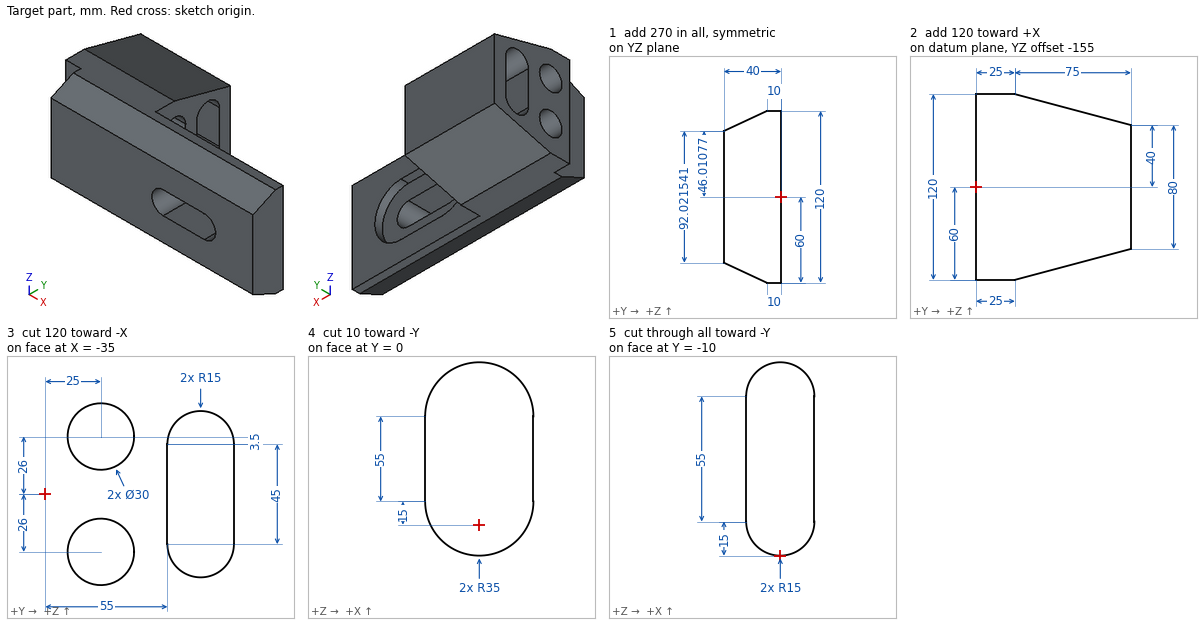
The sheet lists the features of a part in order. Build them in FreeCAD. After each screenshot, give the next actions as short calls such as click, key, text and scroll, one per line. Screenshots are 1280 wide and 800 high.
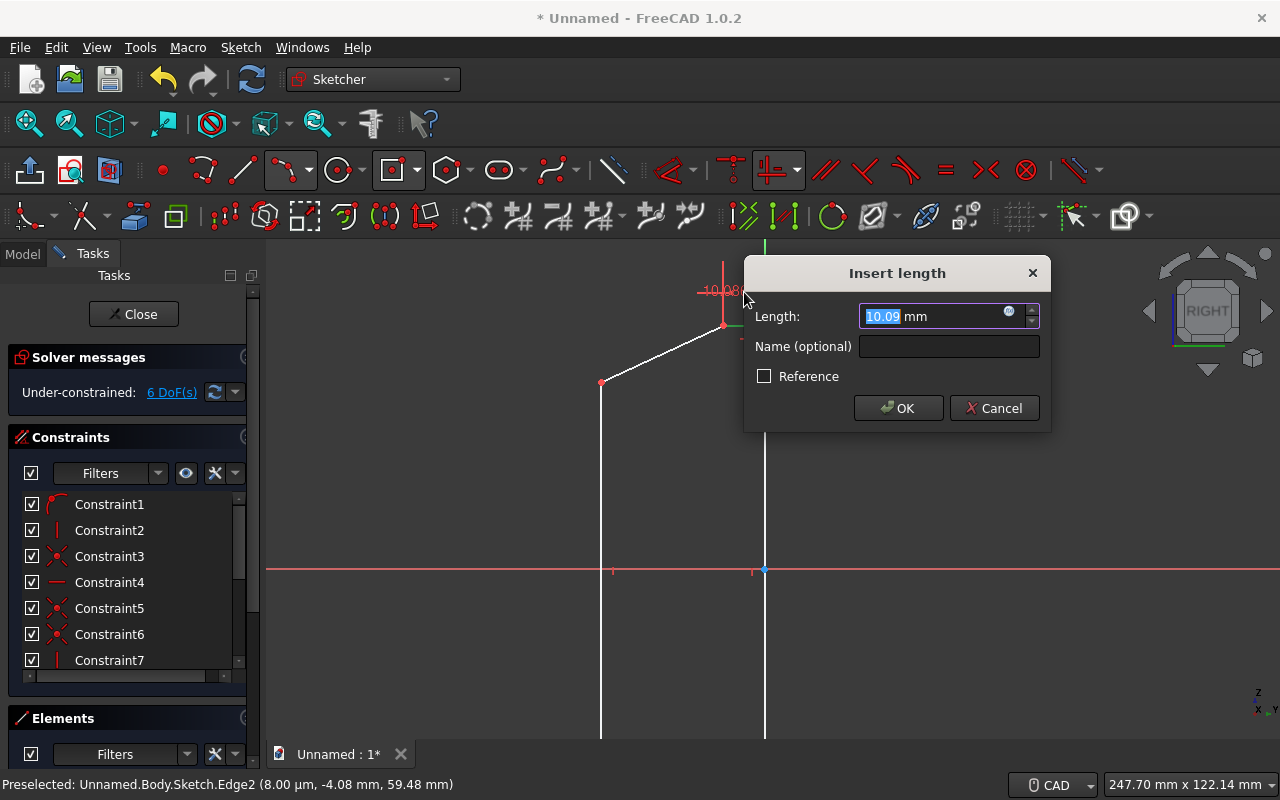
text(10)
key(Return)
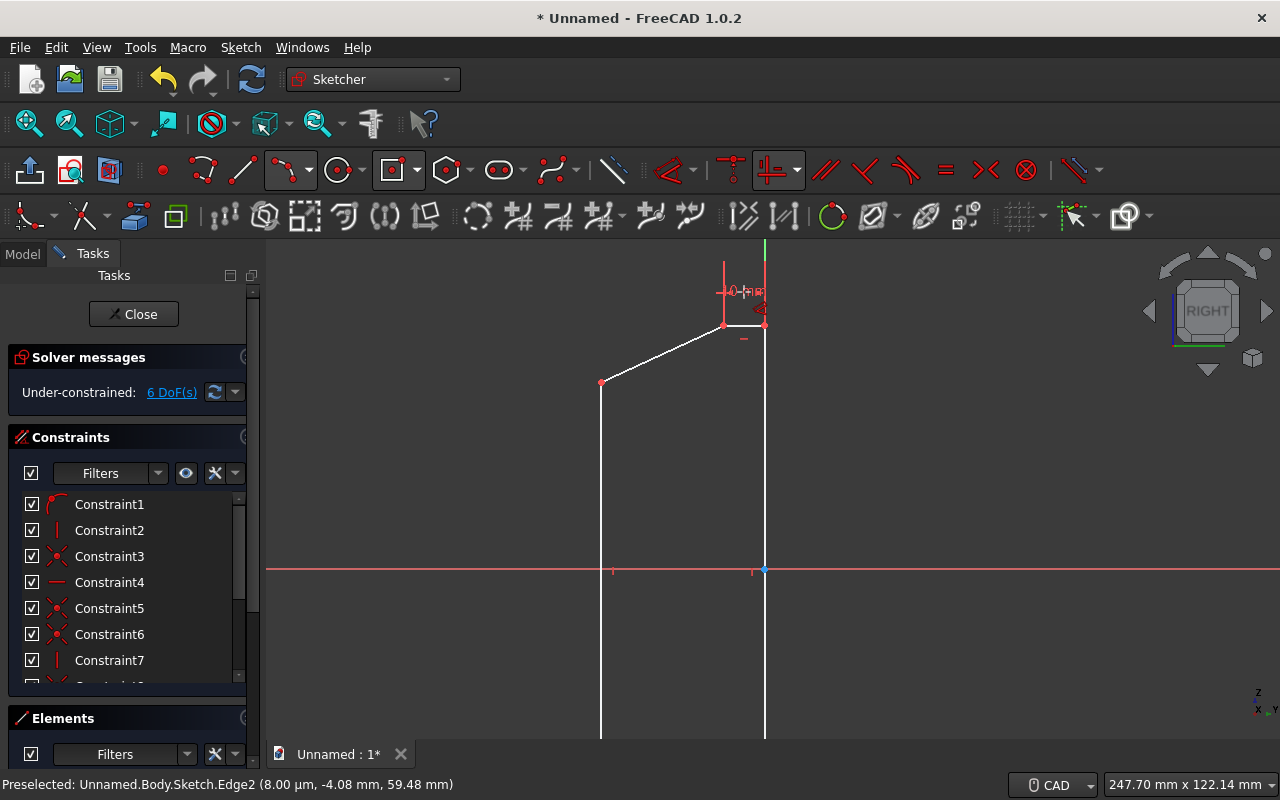
scroll(749, 325, down, 2)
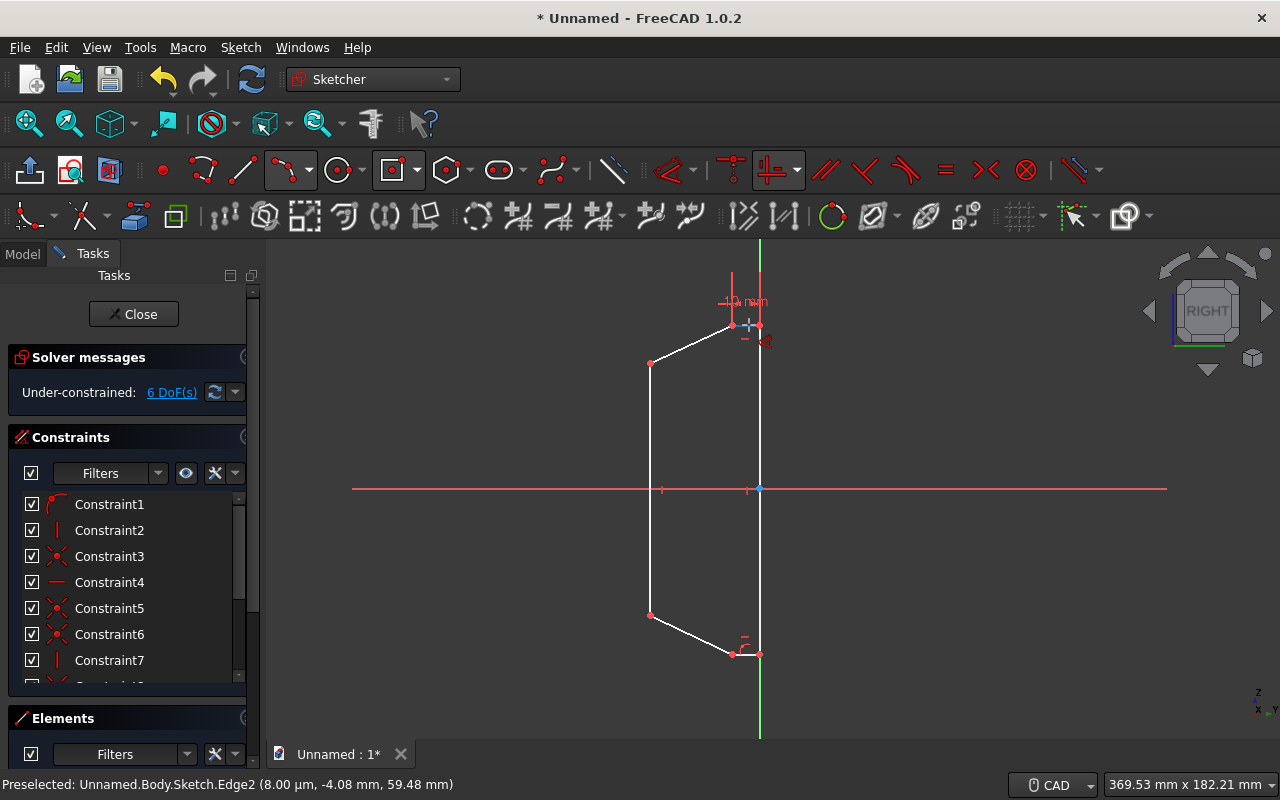
scroll(740, 655, up, 3)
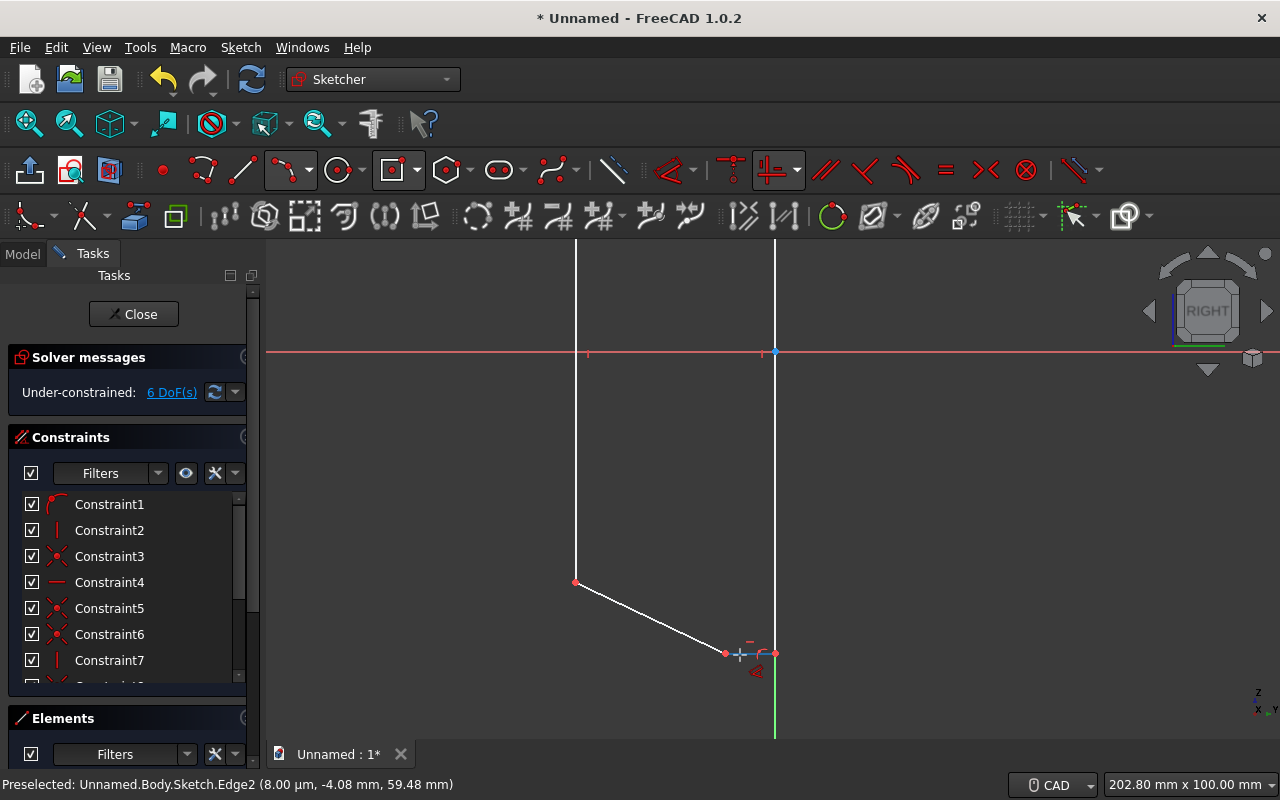
click(740, 654)
click(750, 688)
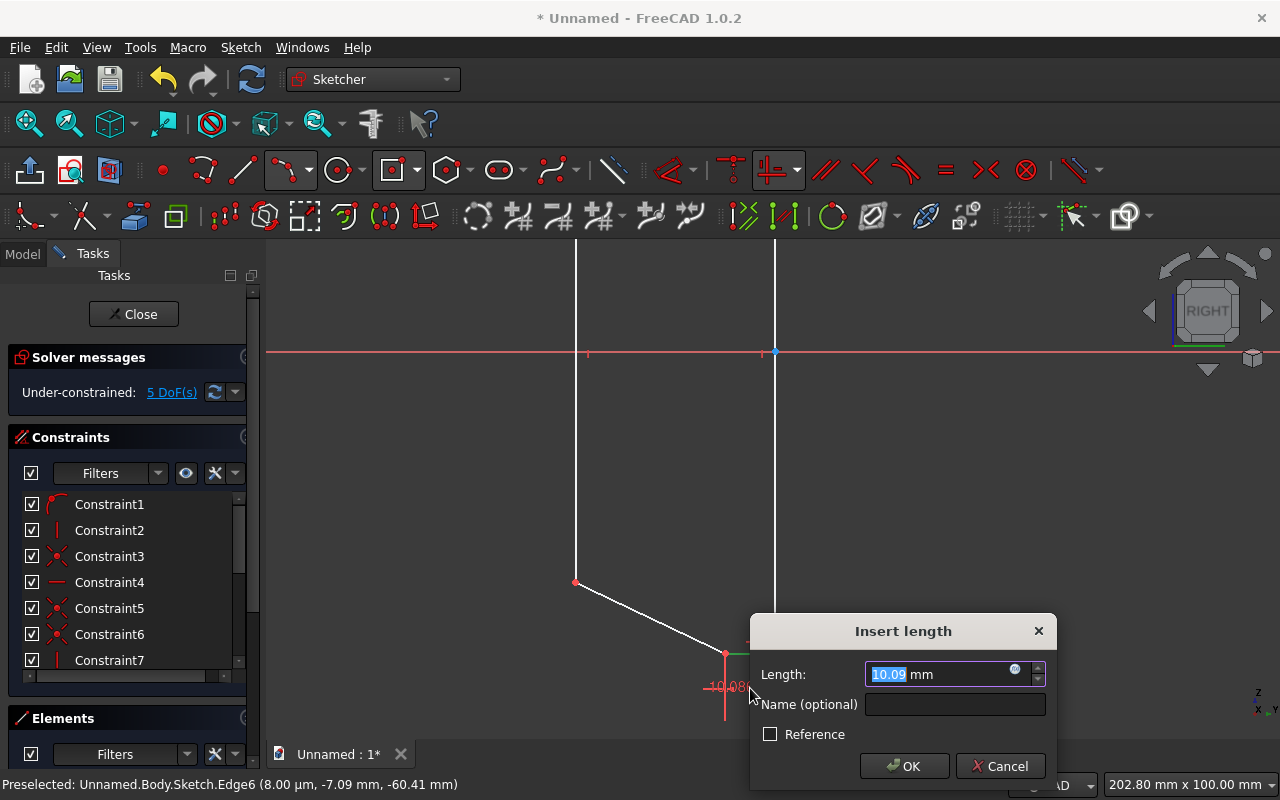
text(10)
key(Return)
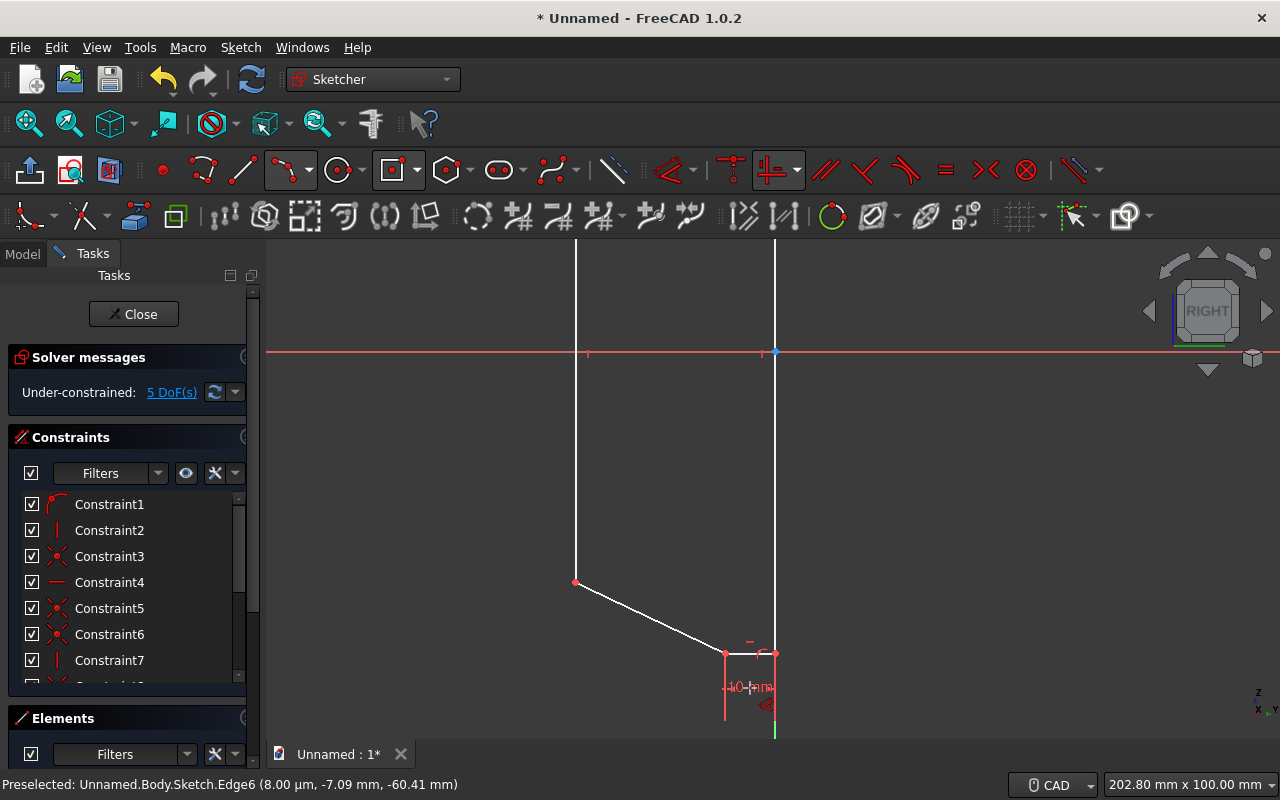
click(775, 474)
click(809, 460)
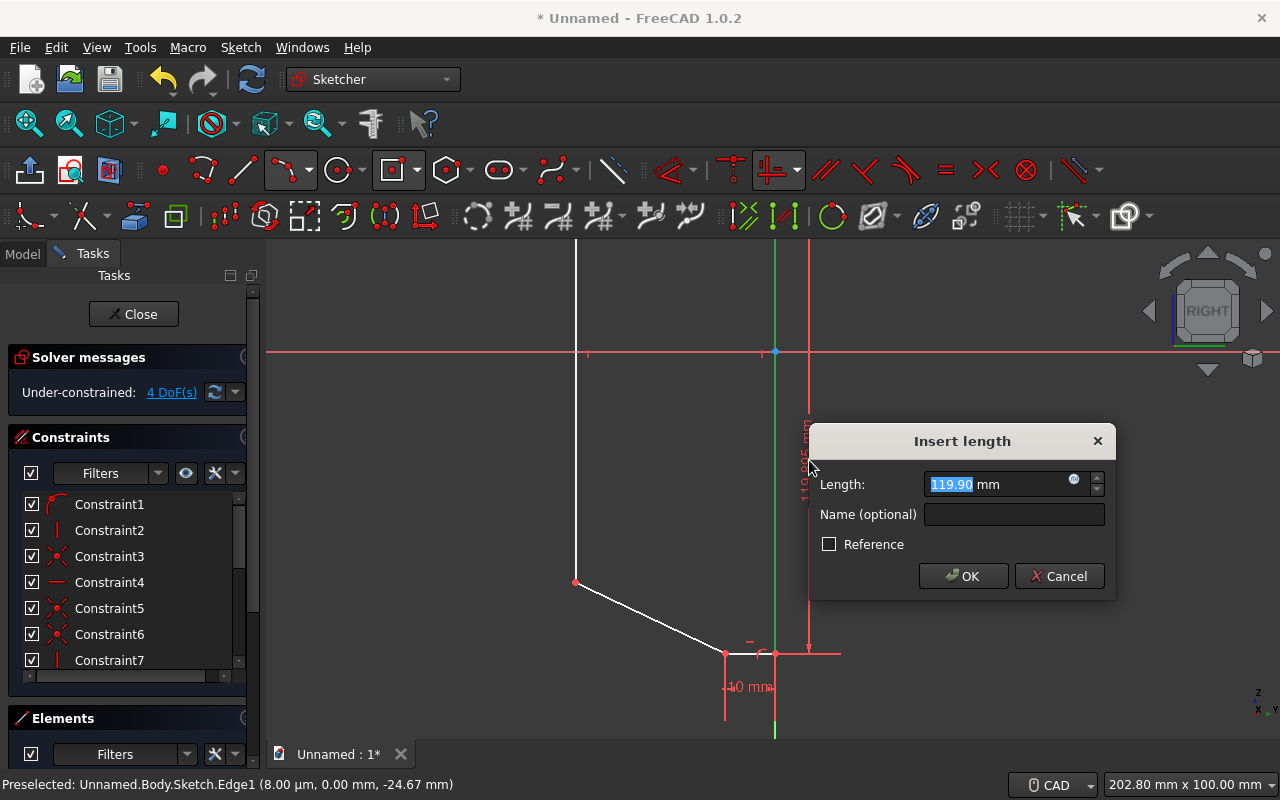
text(120)
key(Return)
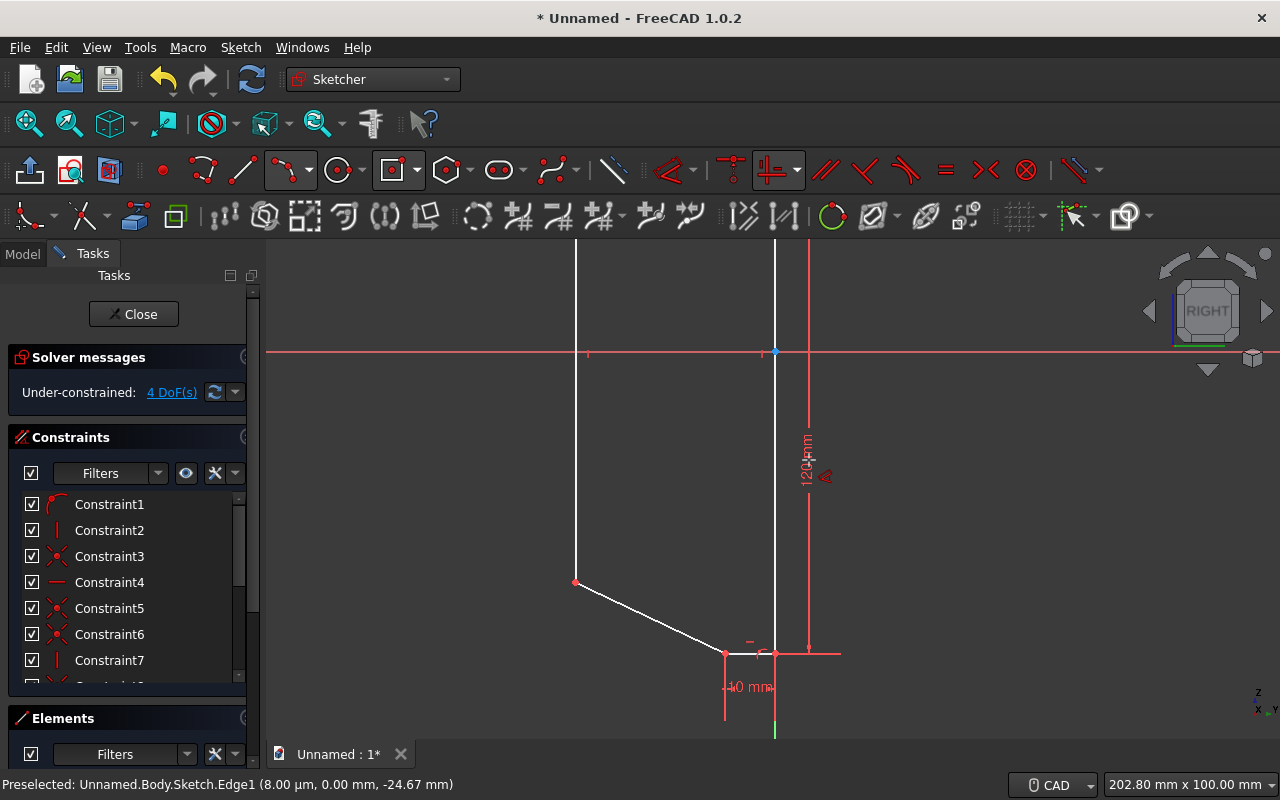
click(775, 654)
click(809, 503)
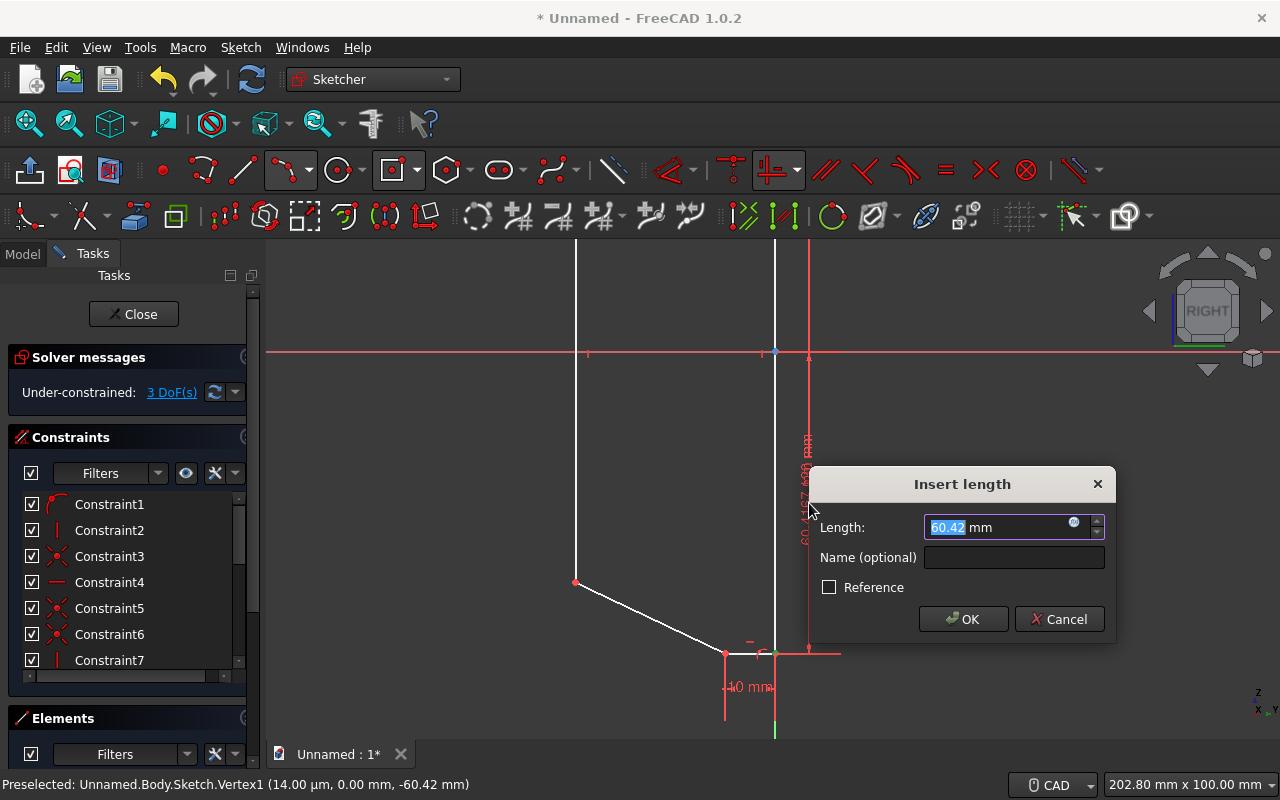
text(60)
key(Return)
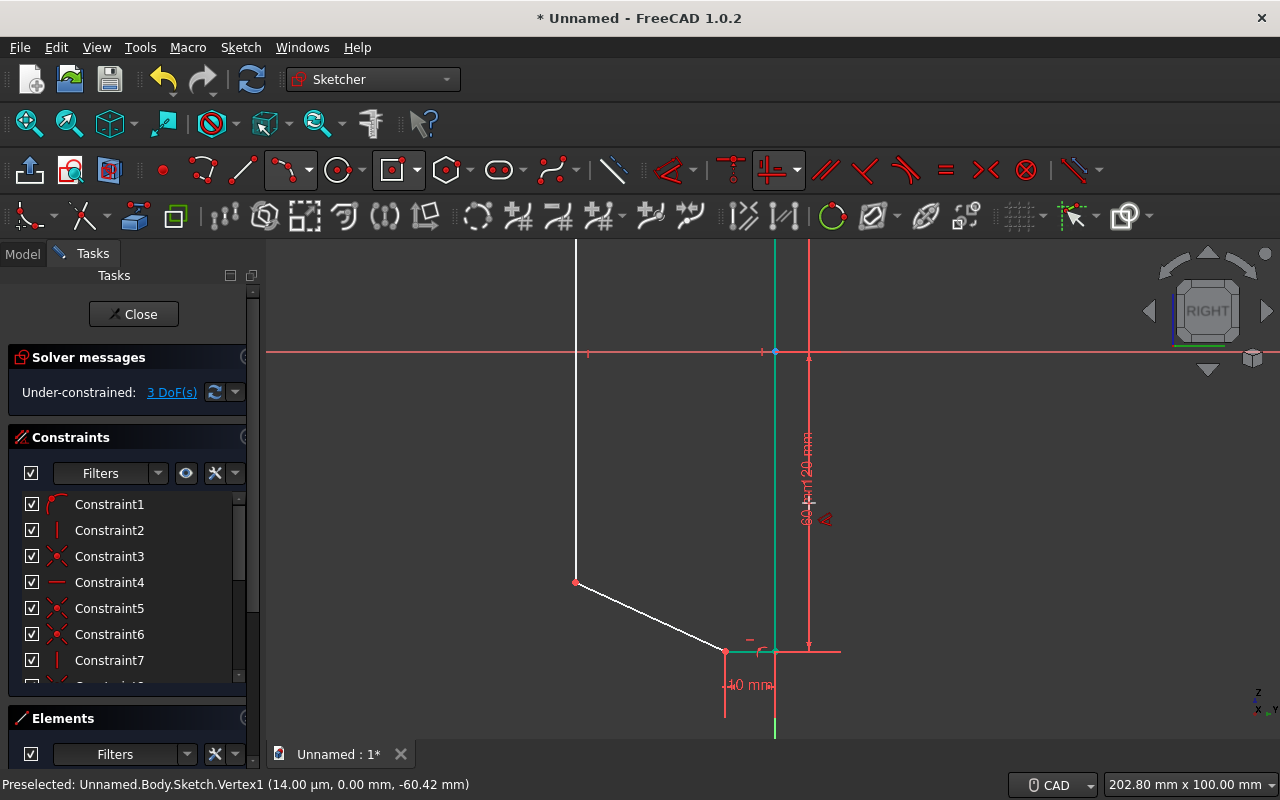
scroll(740, 656, down, 3)